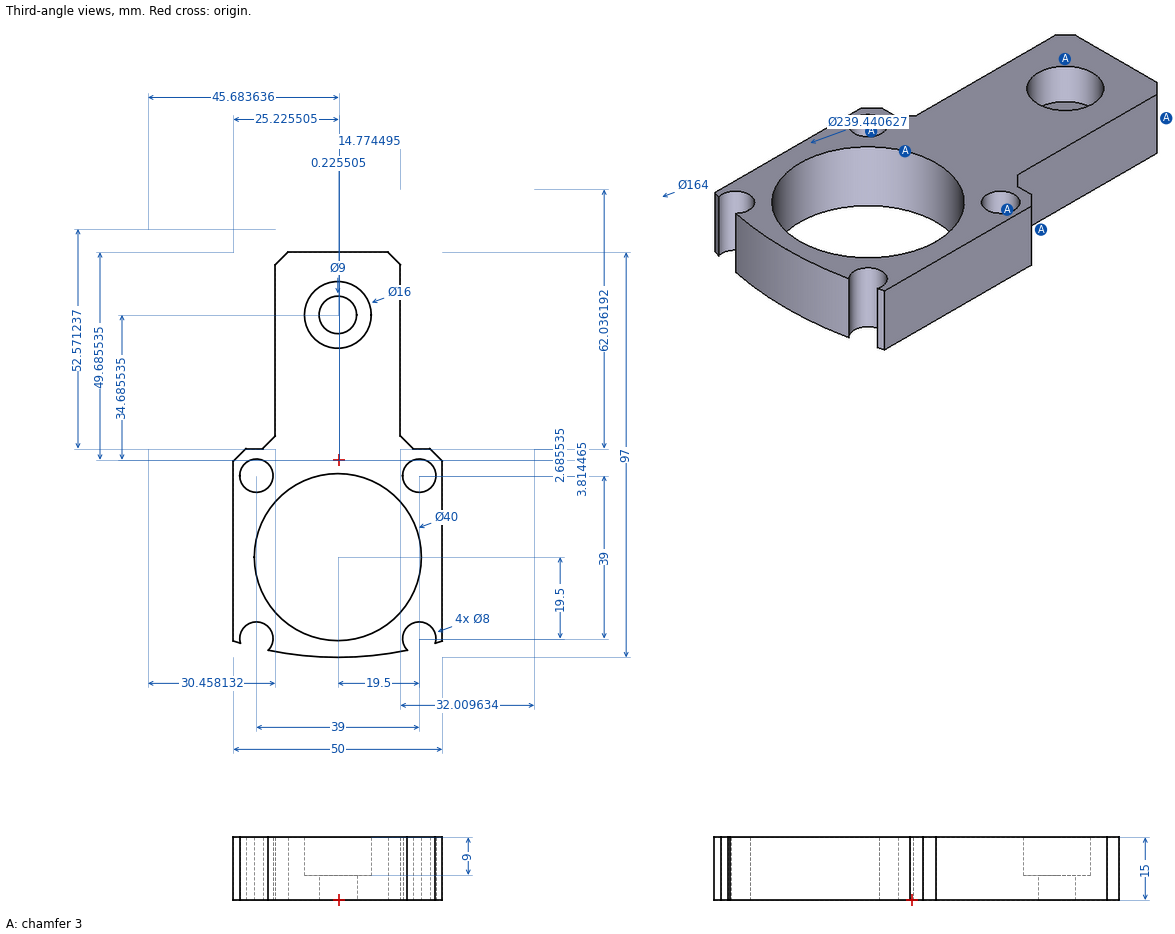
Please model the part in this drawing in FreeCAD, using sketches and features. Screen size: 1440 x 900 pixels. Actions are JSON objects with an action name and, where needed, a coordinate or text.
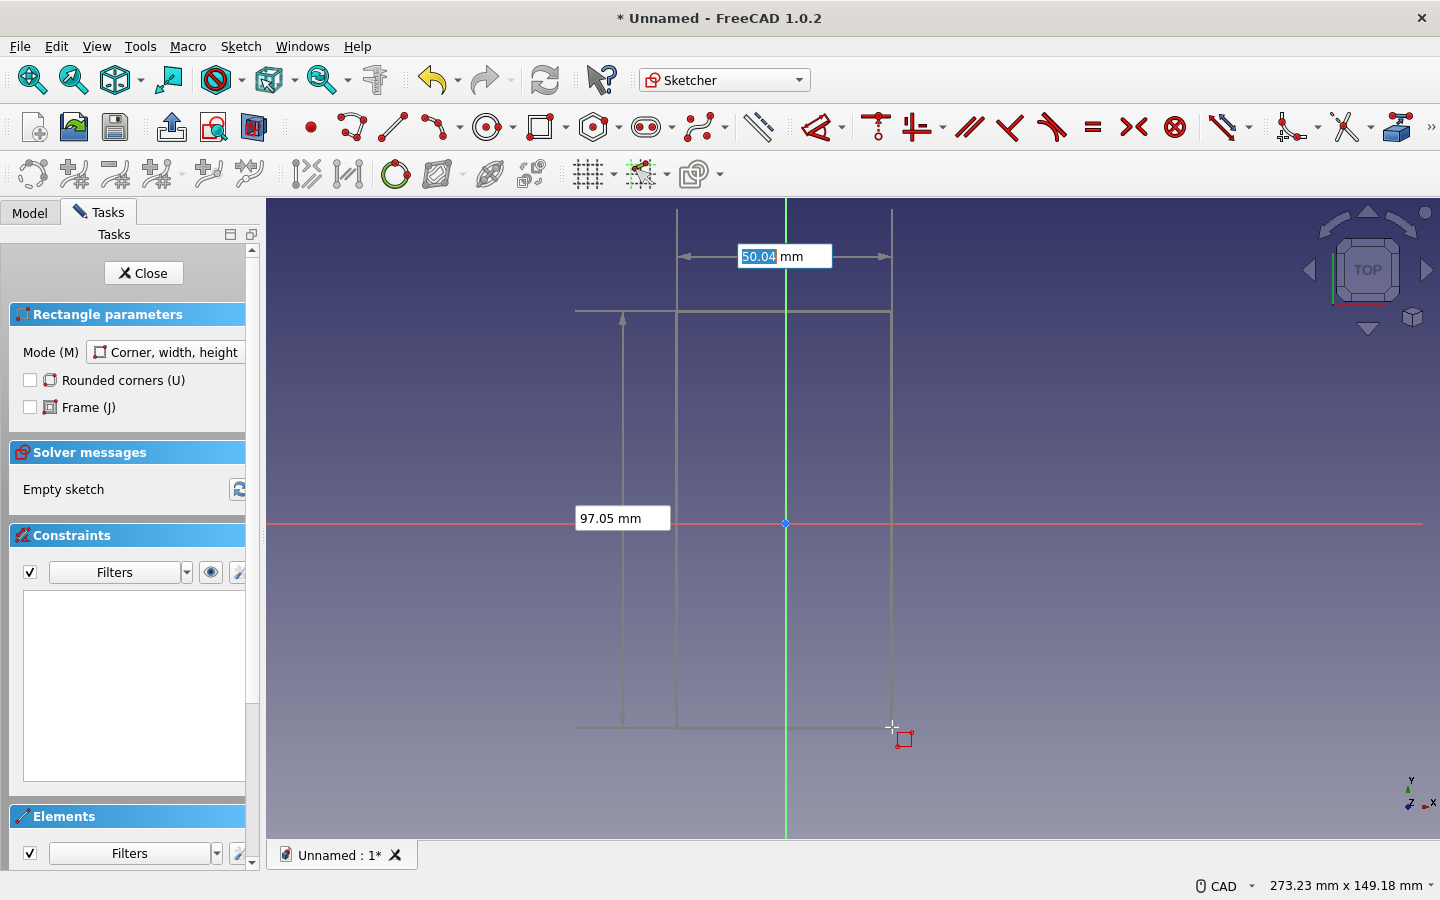
{"action": "type", "text": "50"}
{"action": "key", "text": "Tab"}
{"action": "type", "text": "97"}
{"action": "key", "text": "Return"}
{"action": "key", "text": "Escape"}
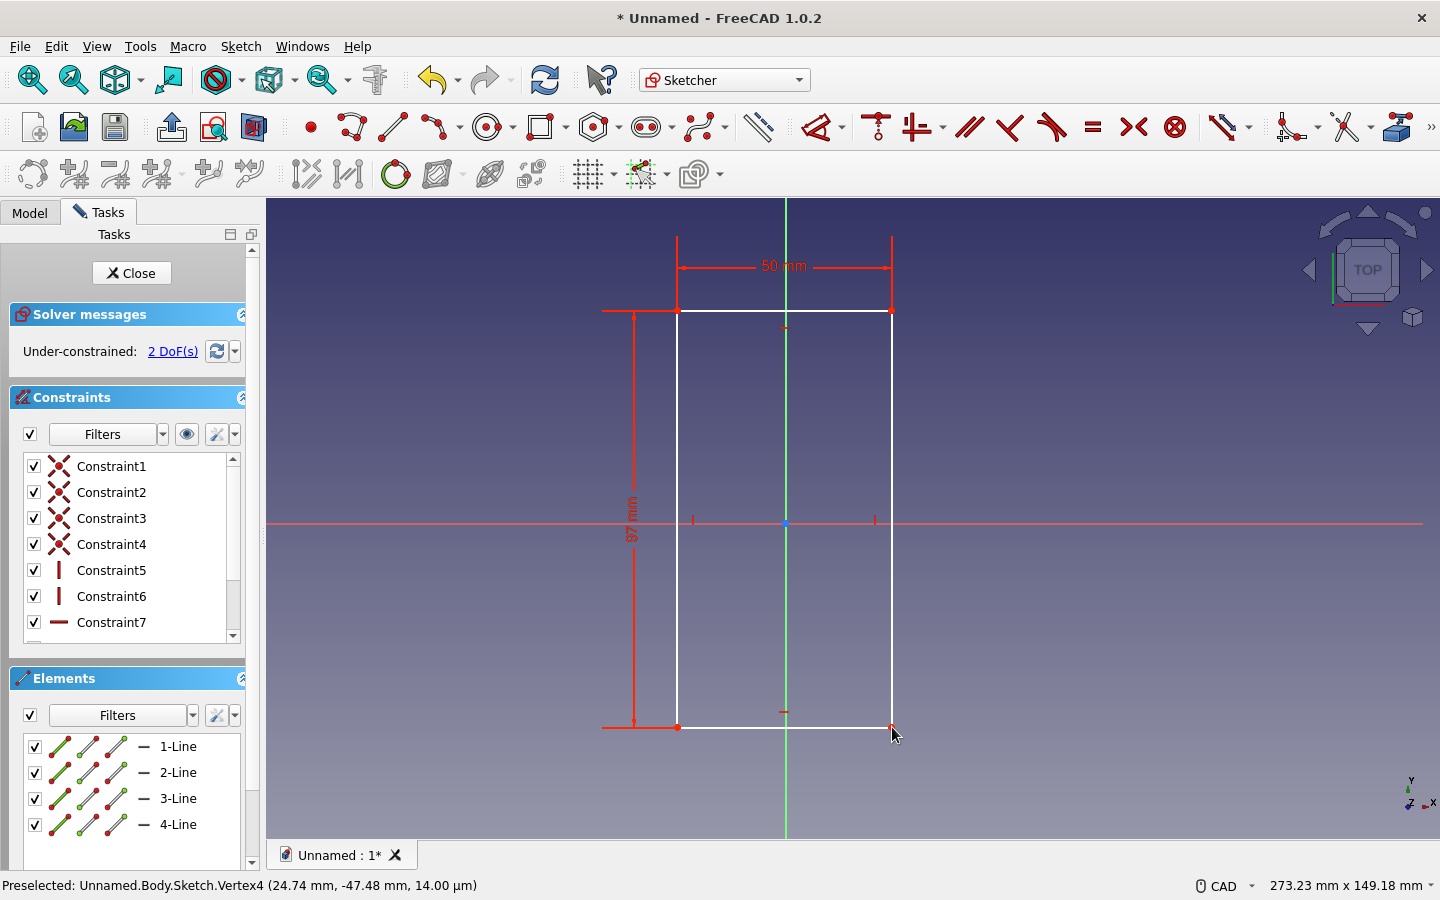
{"action": "left_click", "coordinate": [816, 128]}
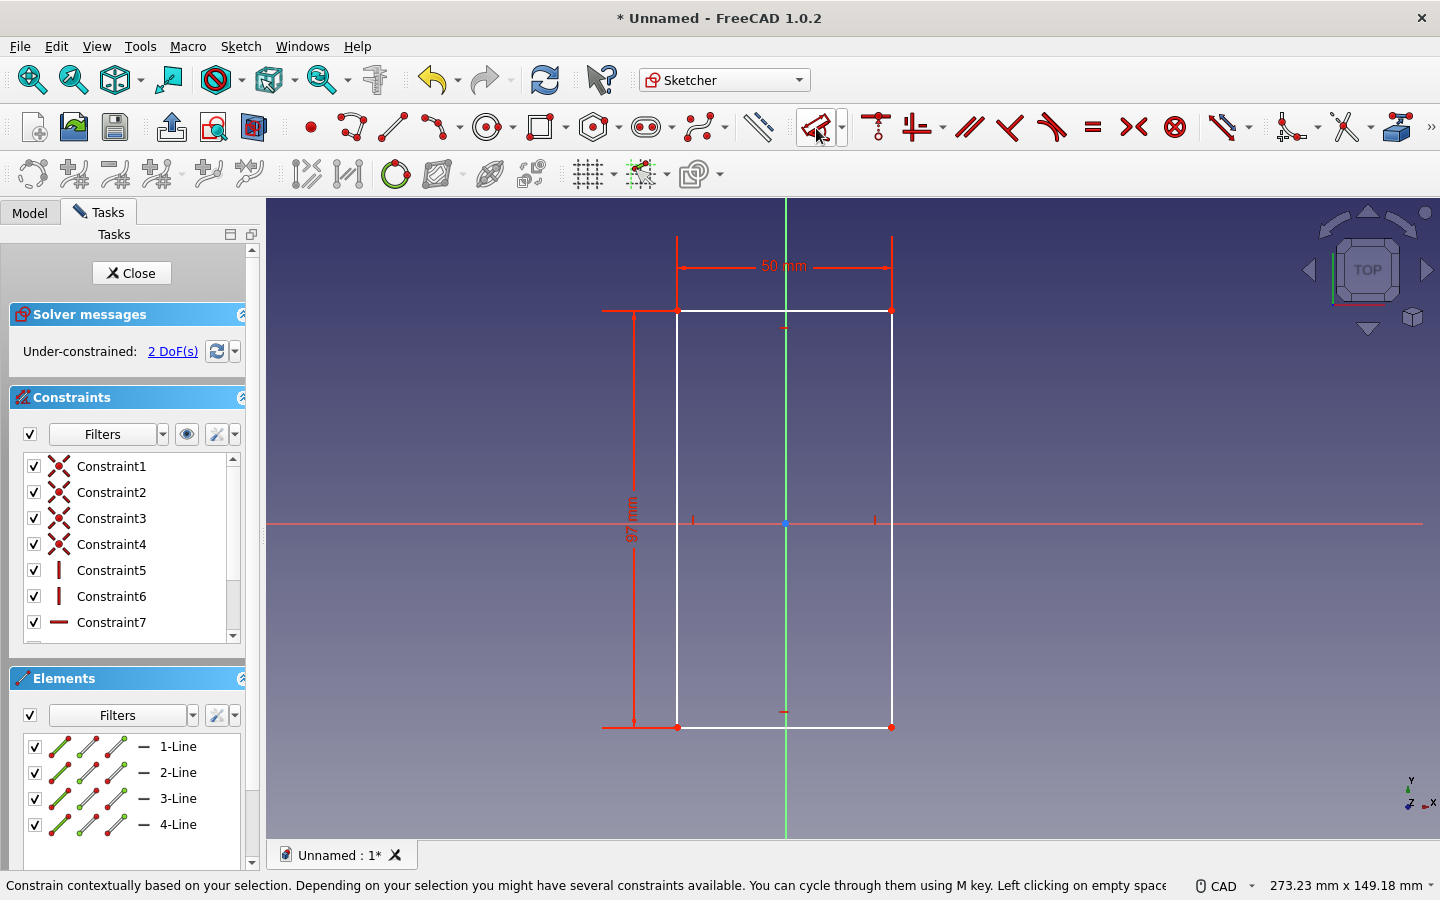
{"action": "left_click", "coordinate": [677, 311]}
{"action": "left_click", "coordinate": [731, 277]}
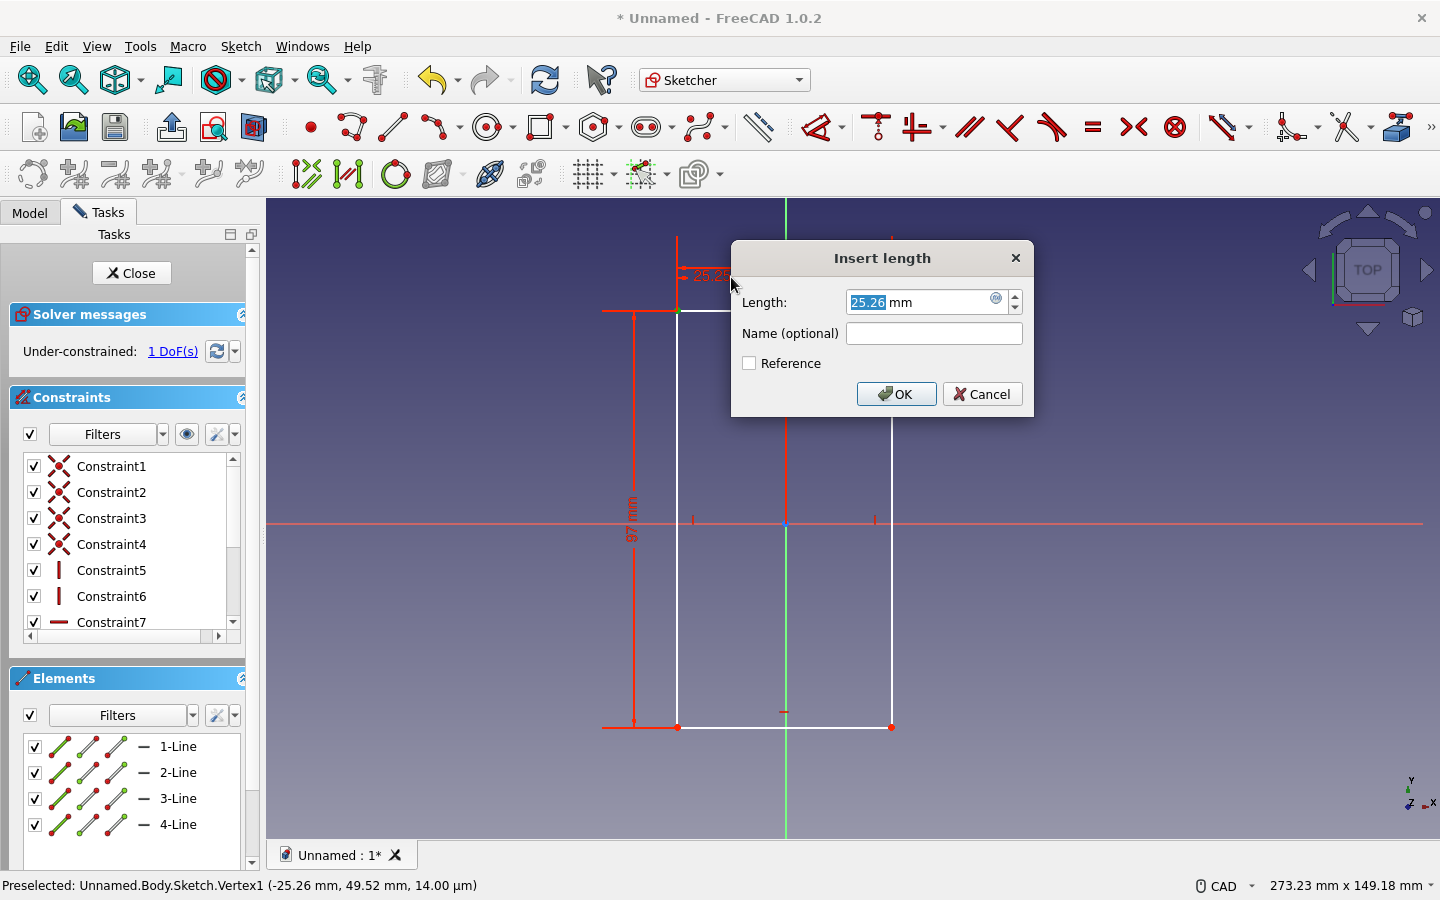
{"action": "type", "text": "25.225505"}
{"action": "key", "text": "Return"}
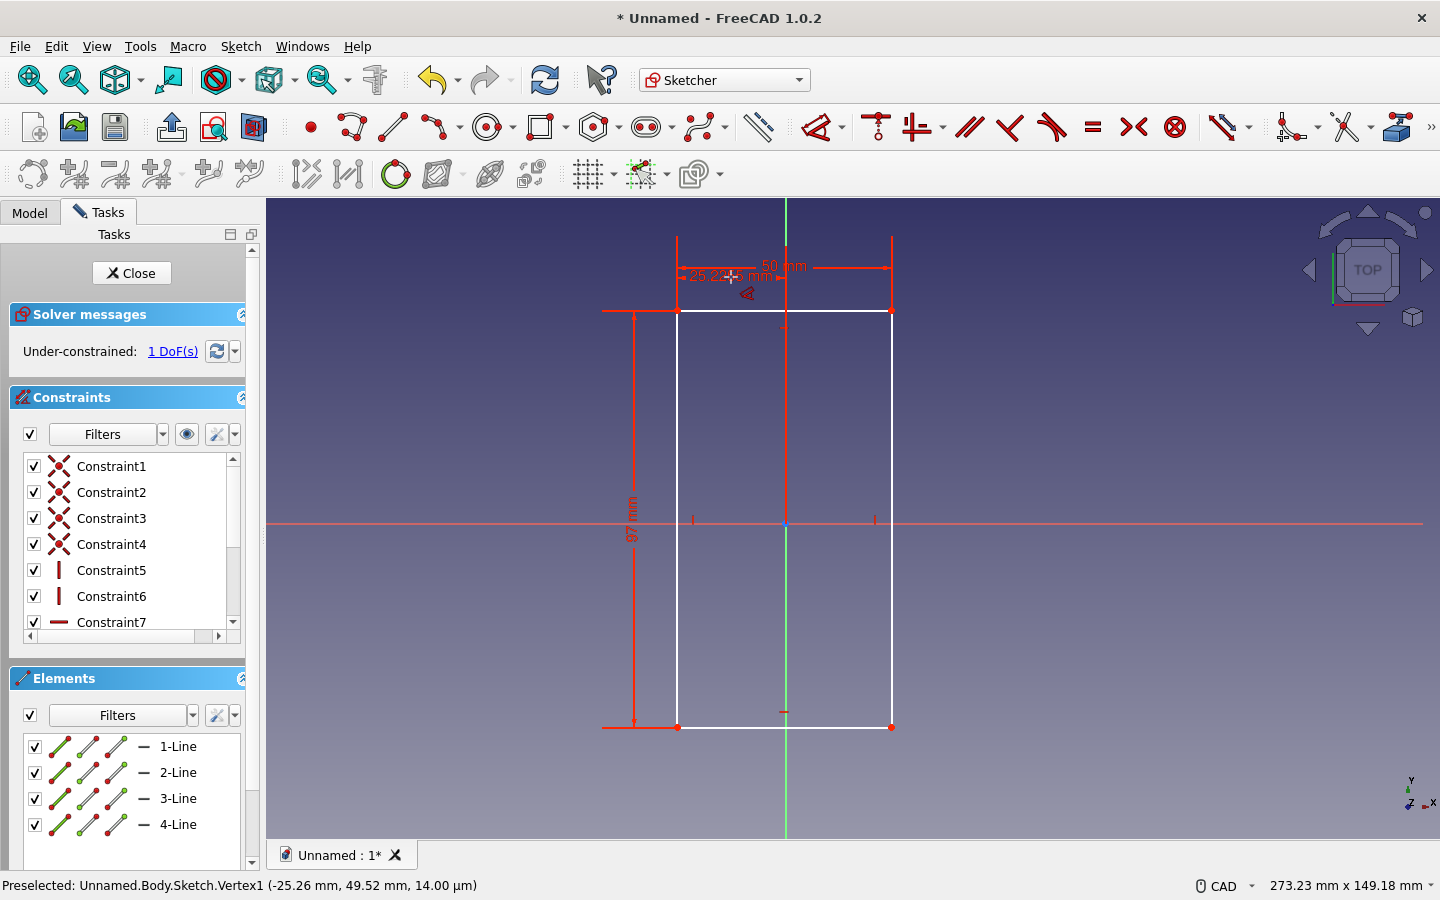
{"action": "left_click", "coordinate": [677, 311]}
{"action": "left_click", "coordinate": [643, 417]}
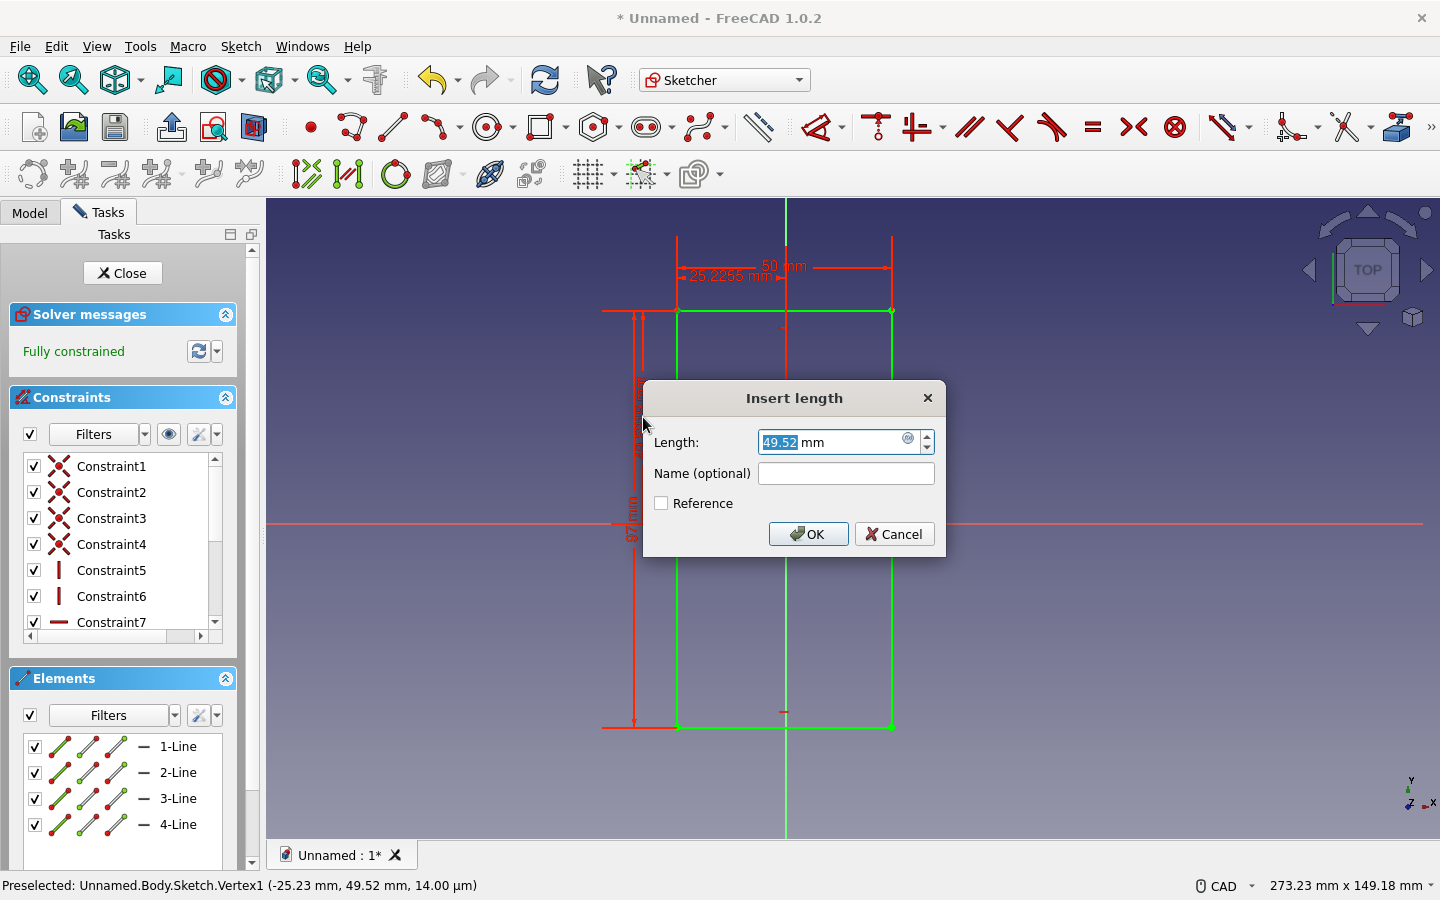
{"action": "type", "text": "49.685535"}
{"action": "key", "text": "Return"}
{"action": "key", "text": "Escape"}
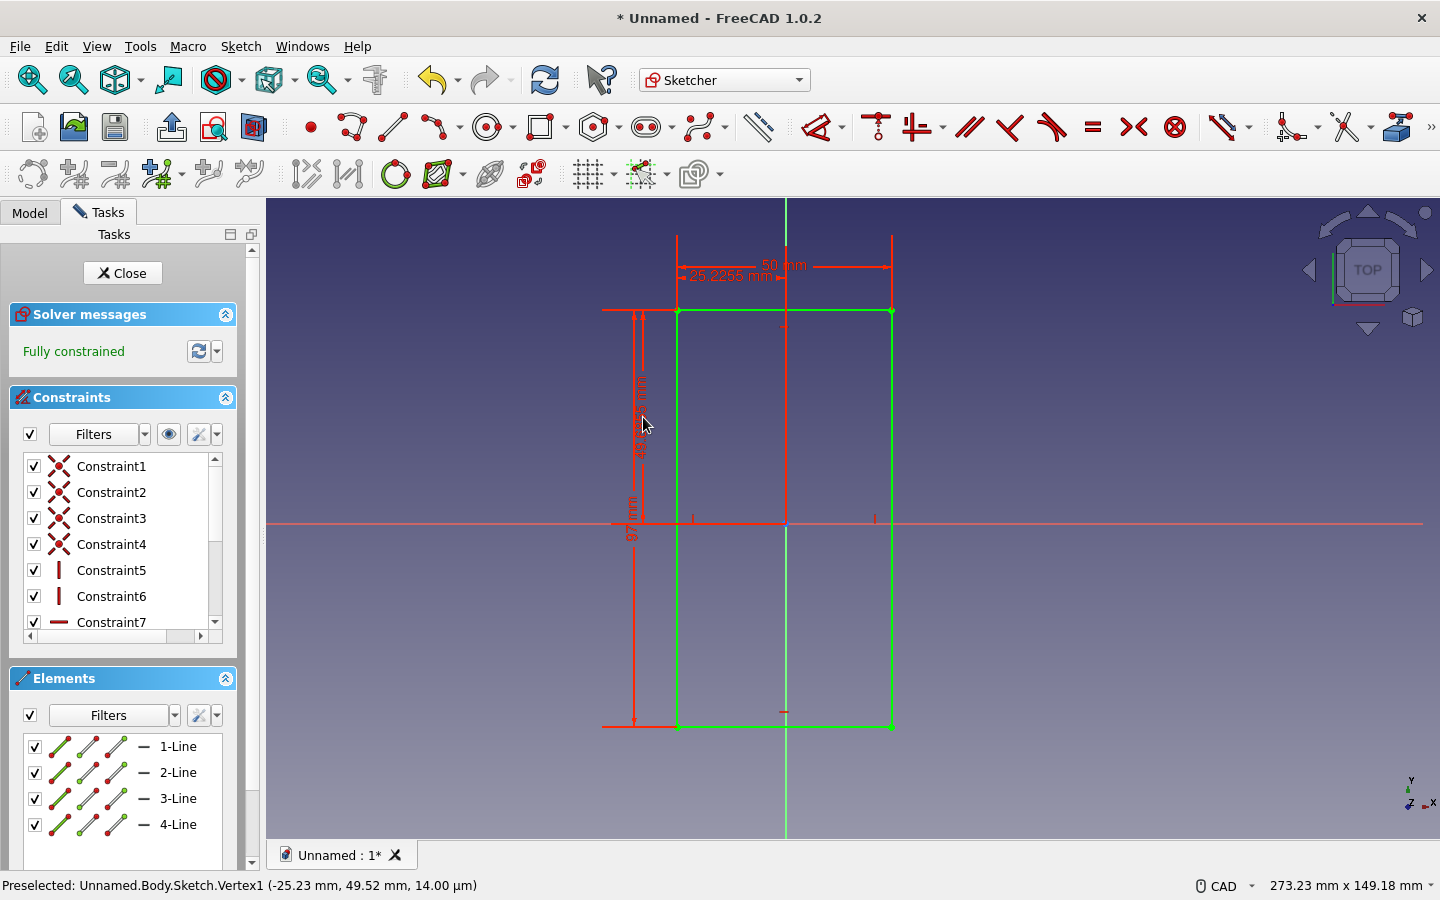
{"action": "left_click", "coordinate": [123, 273]}